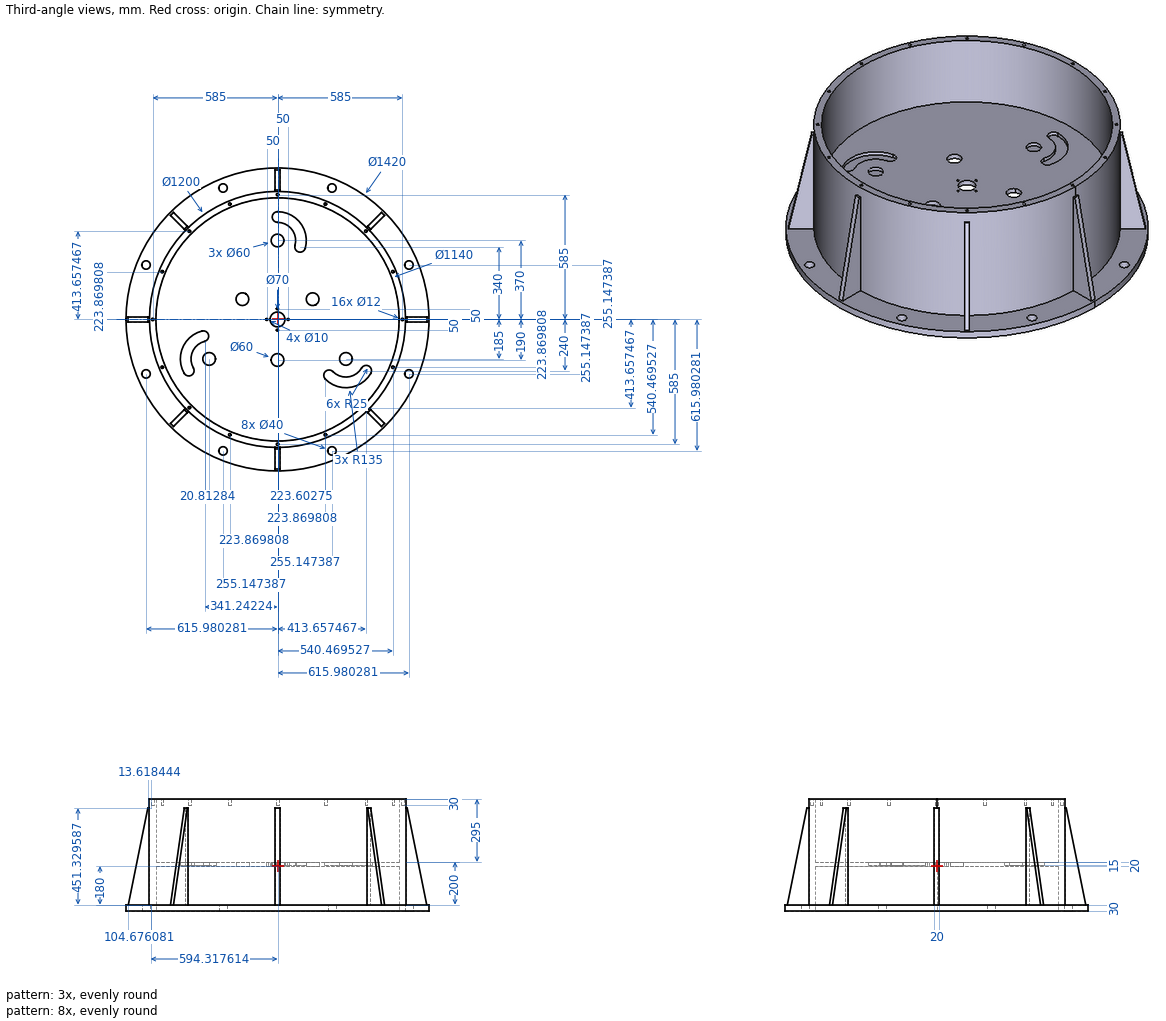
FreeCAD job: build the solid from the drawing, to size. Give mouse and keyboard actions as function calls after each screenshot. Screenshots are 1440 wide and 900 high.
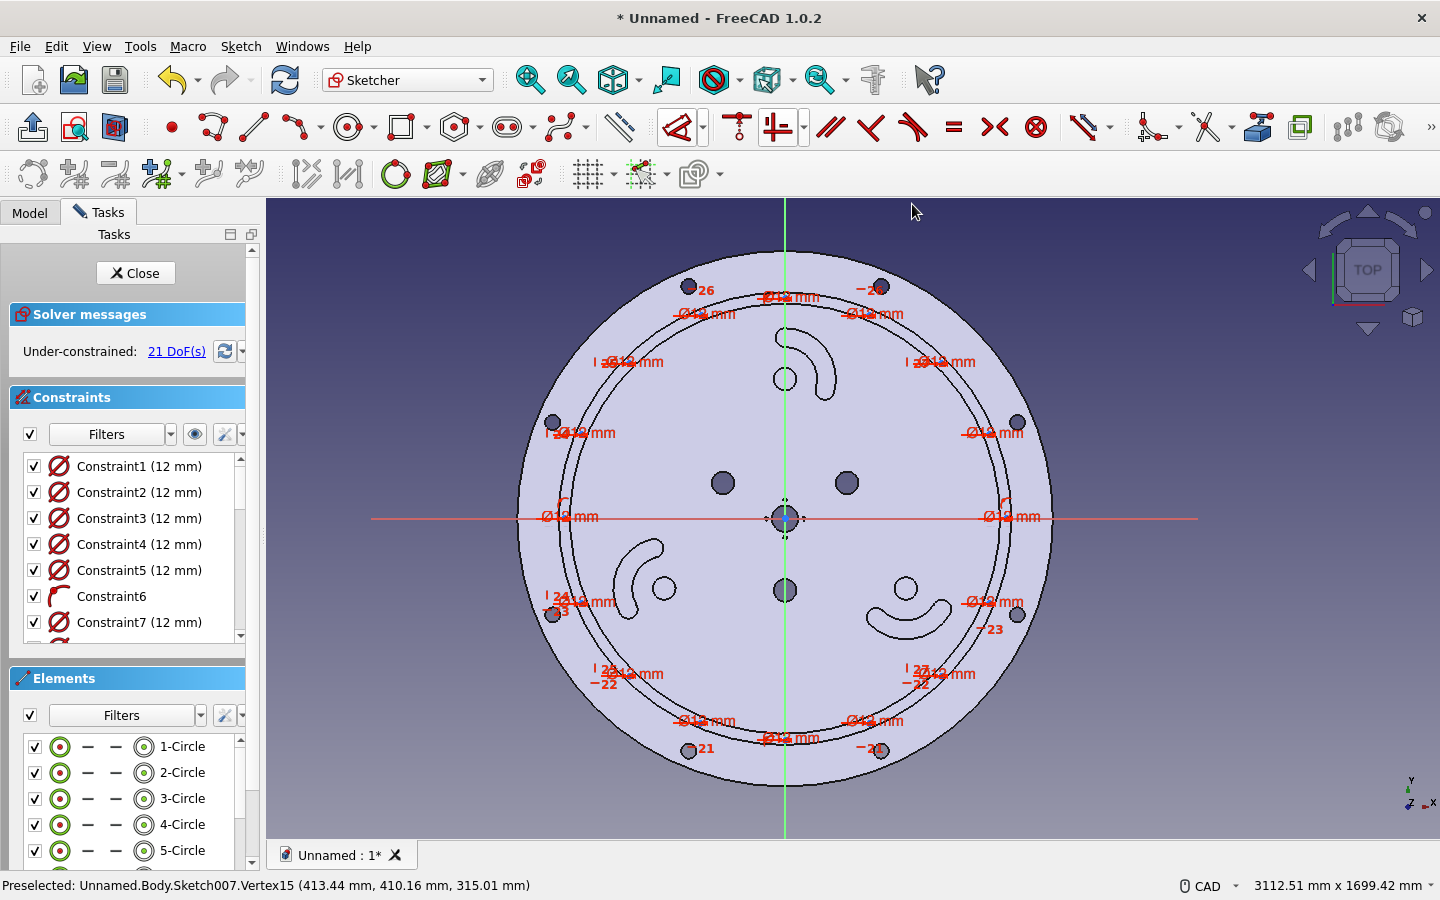
click(989, 604)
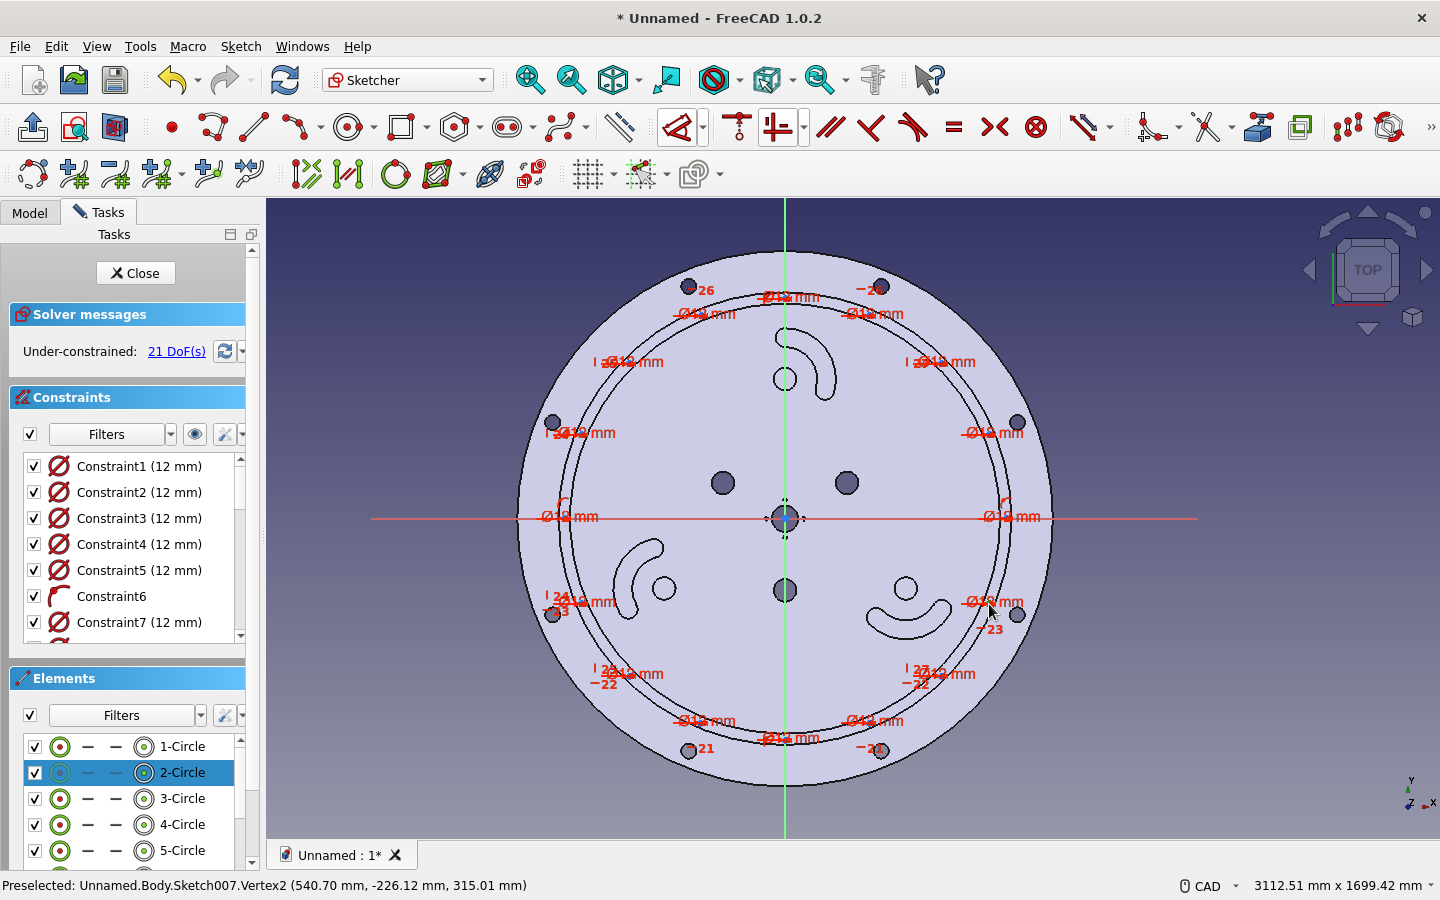
click(989, 435)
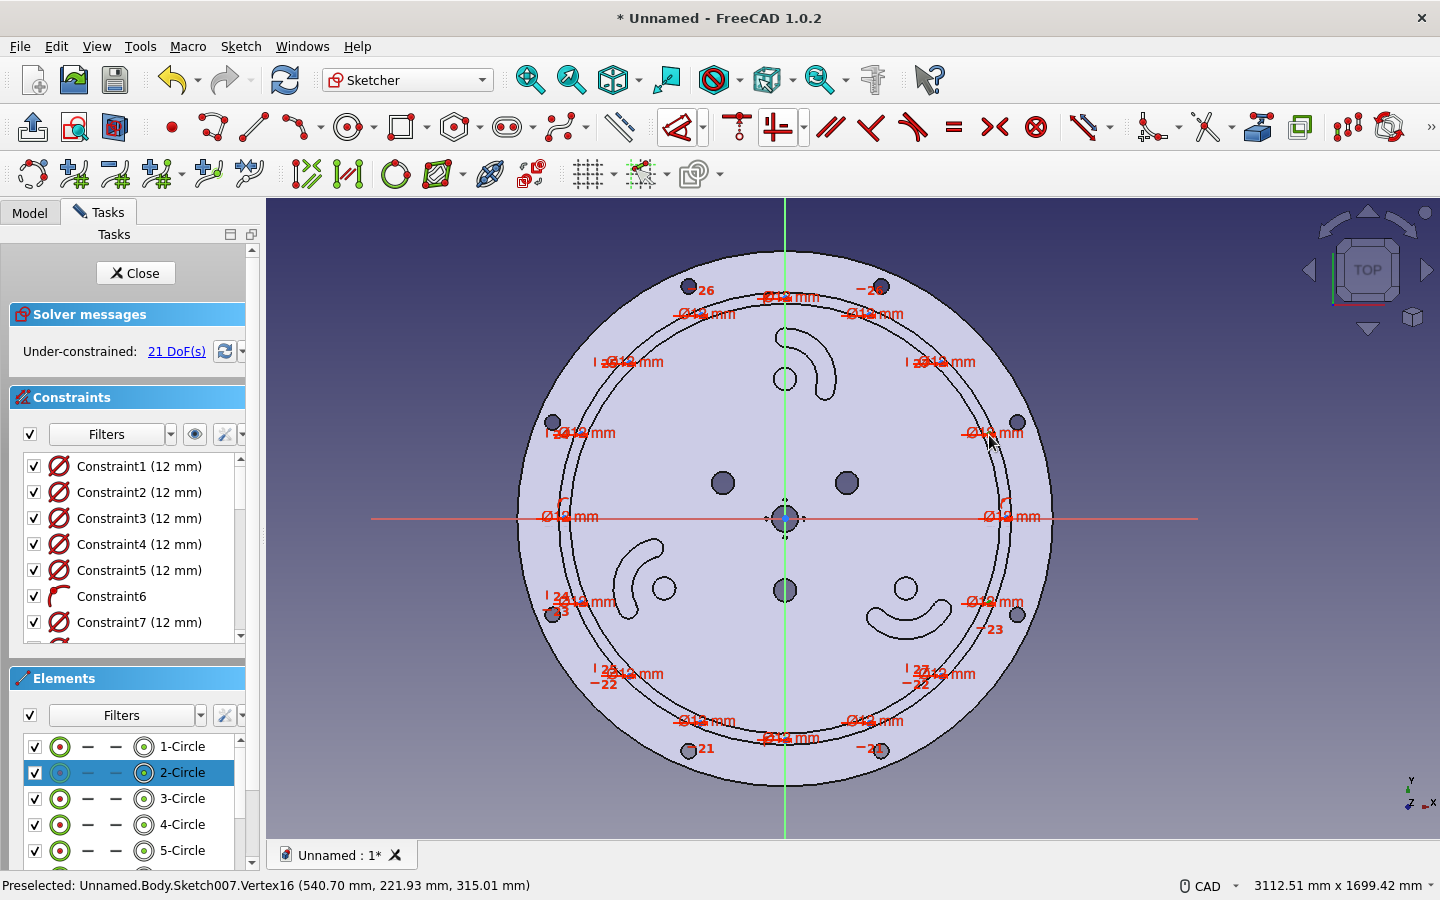
click(804, 128)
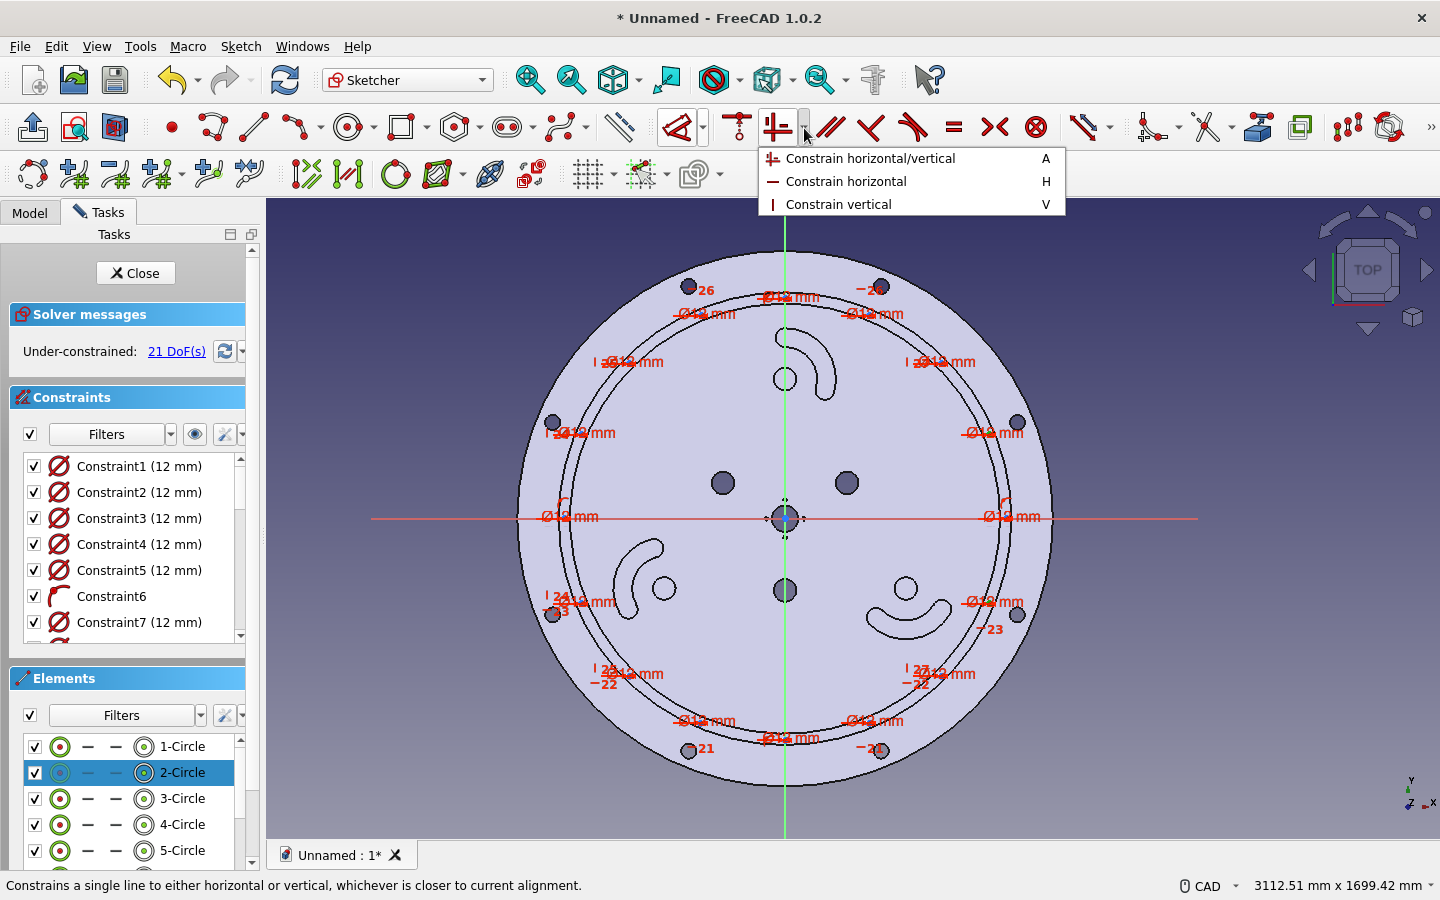
click(912, 204)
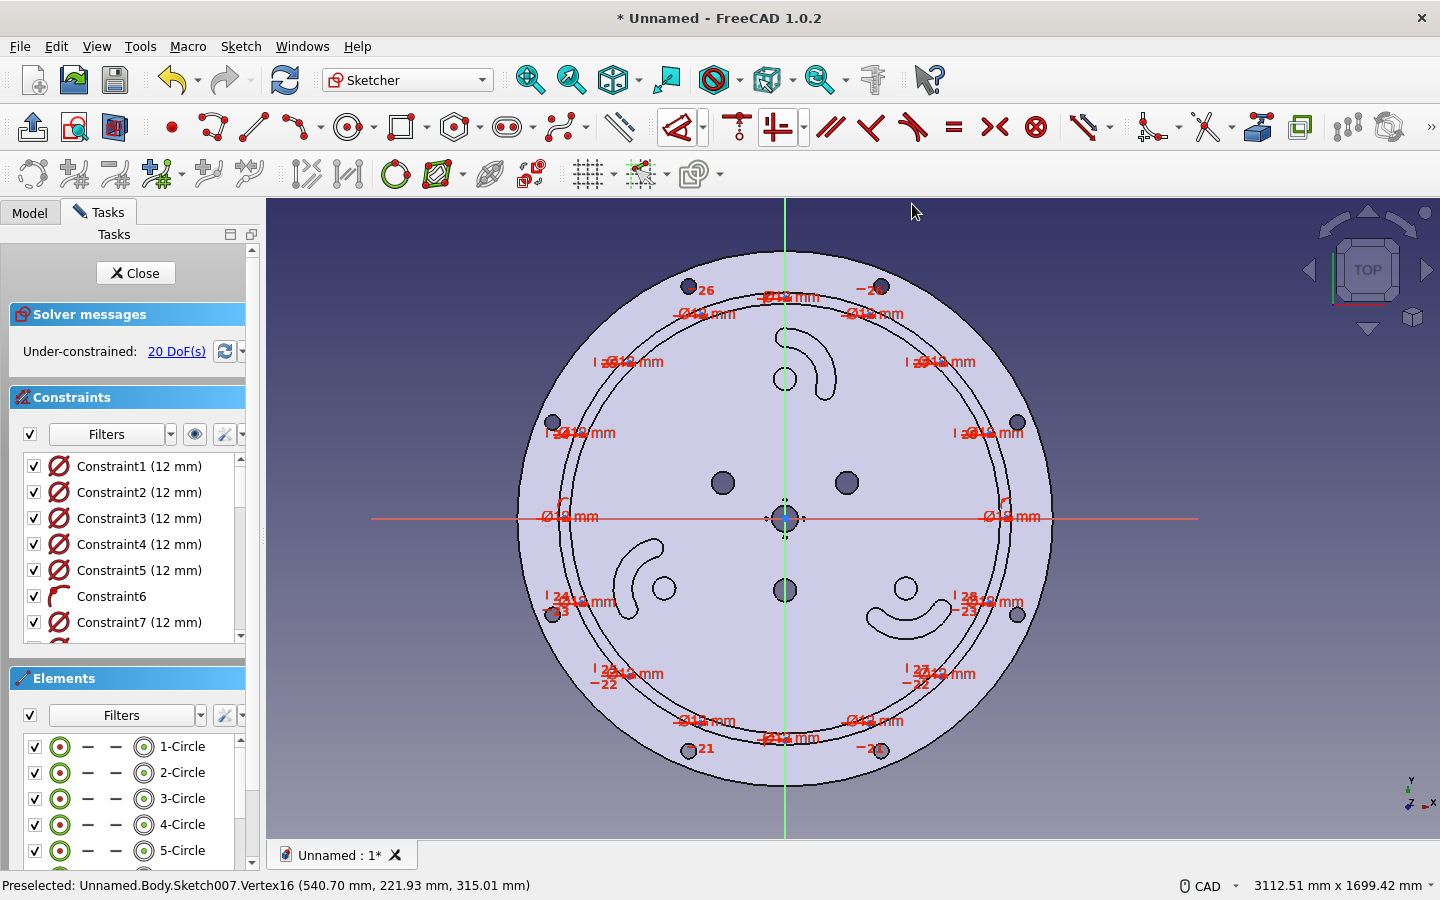
click(701, 723)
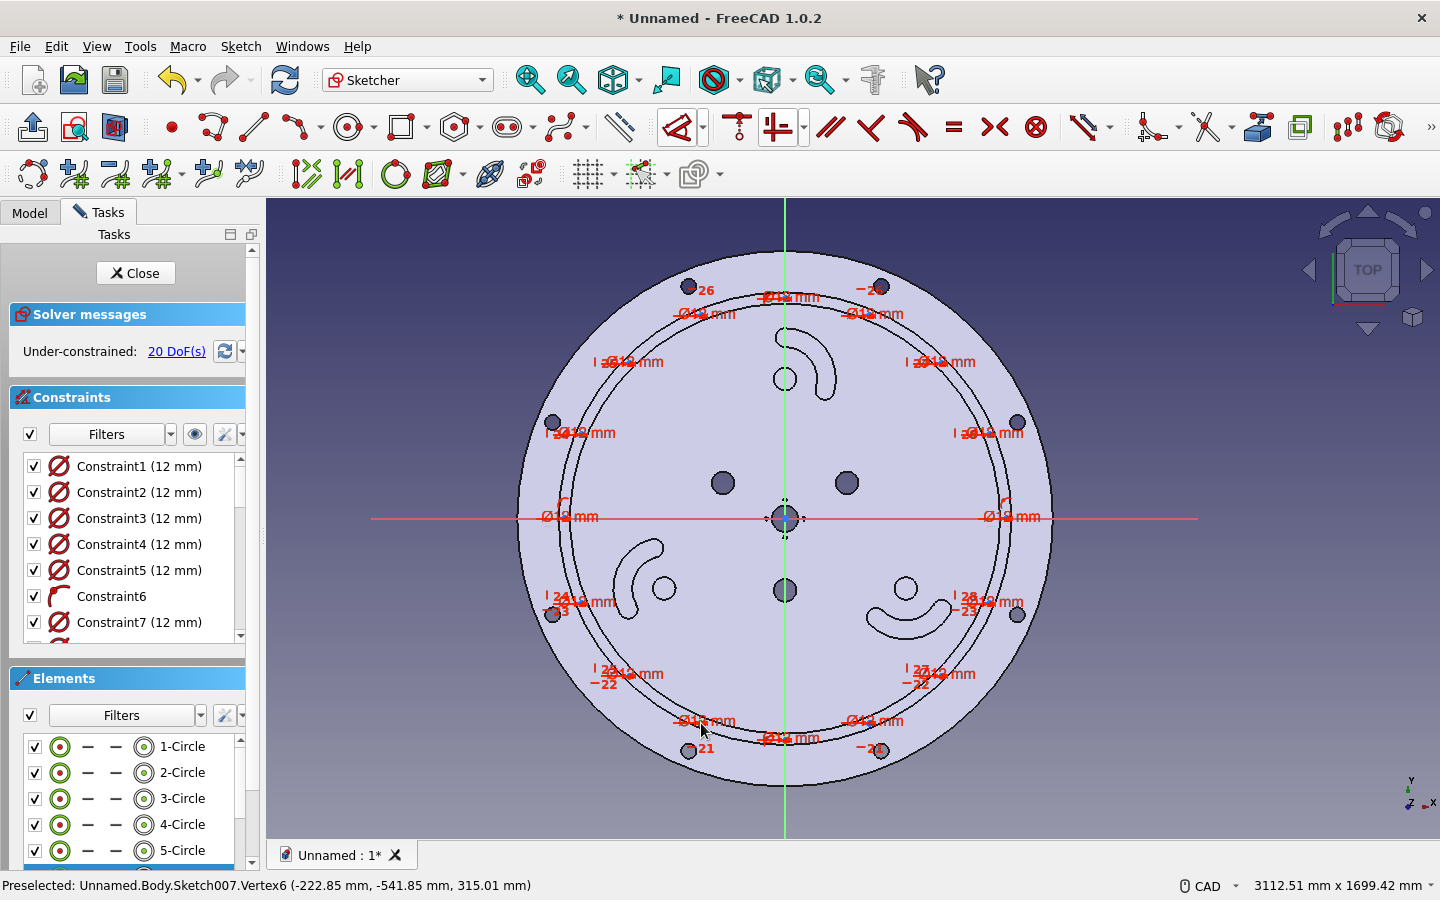
click(701, 316)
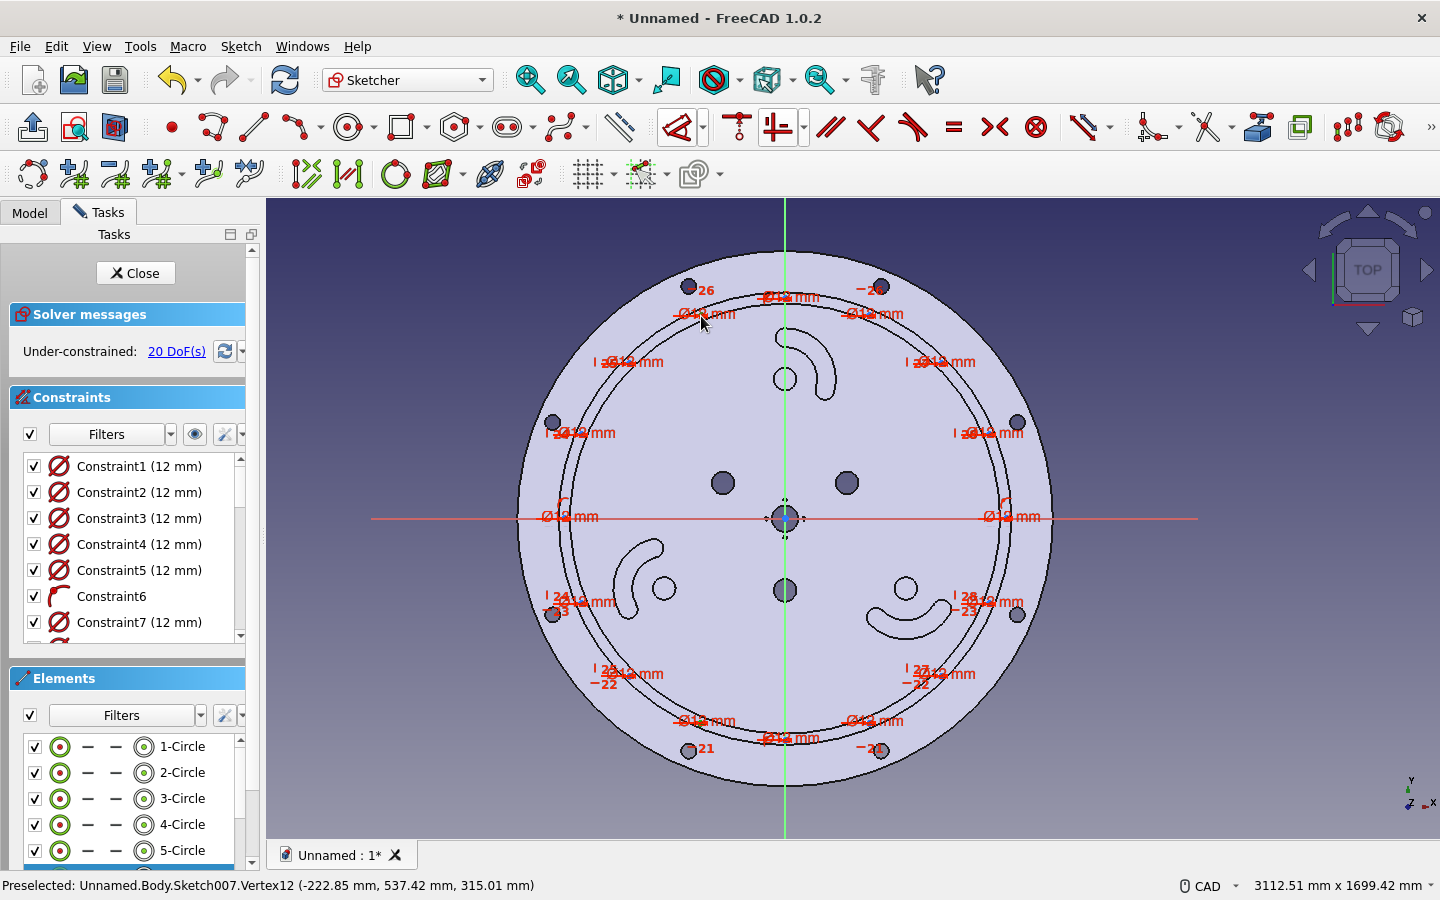
click(434, 519)